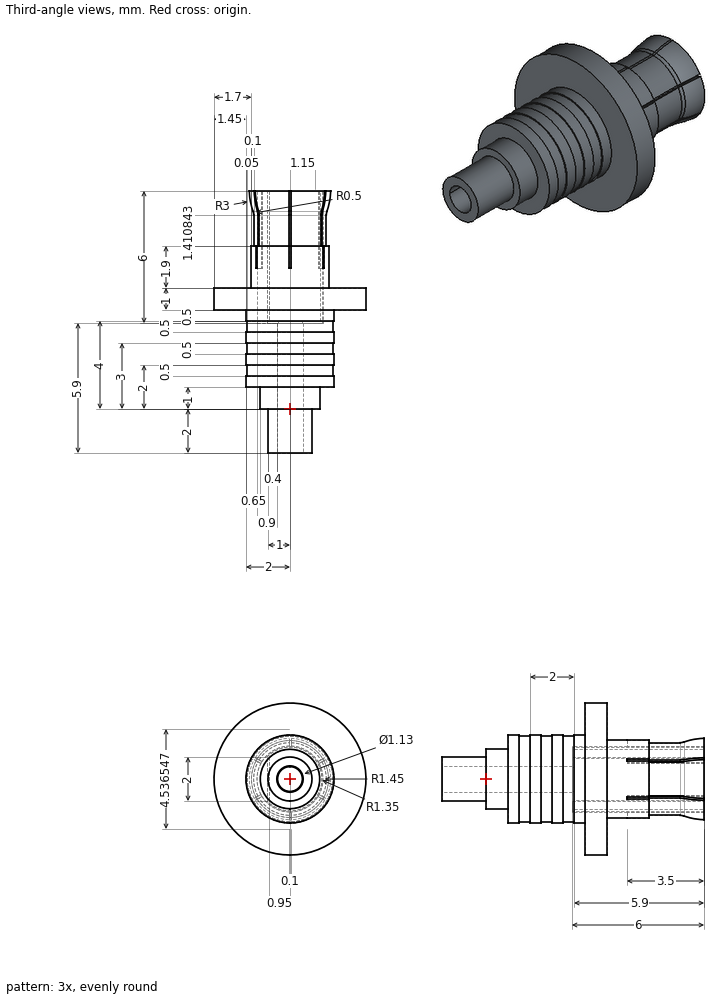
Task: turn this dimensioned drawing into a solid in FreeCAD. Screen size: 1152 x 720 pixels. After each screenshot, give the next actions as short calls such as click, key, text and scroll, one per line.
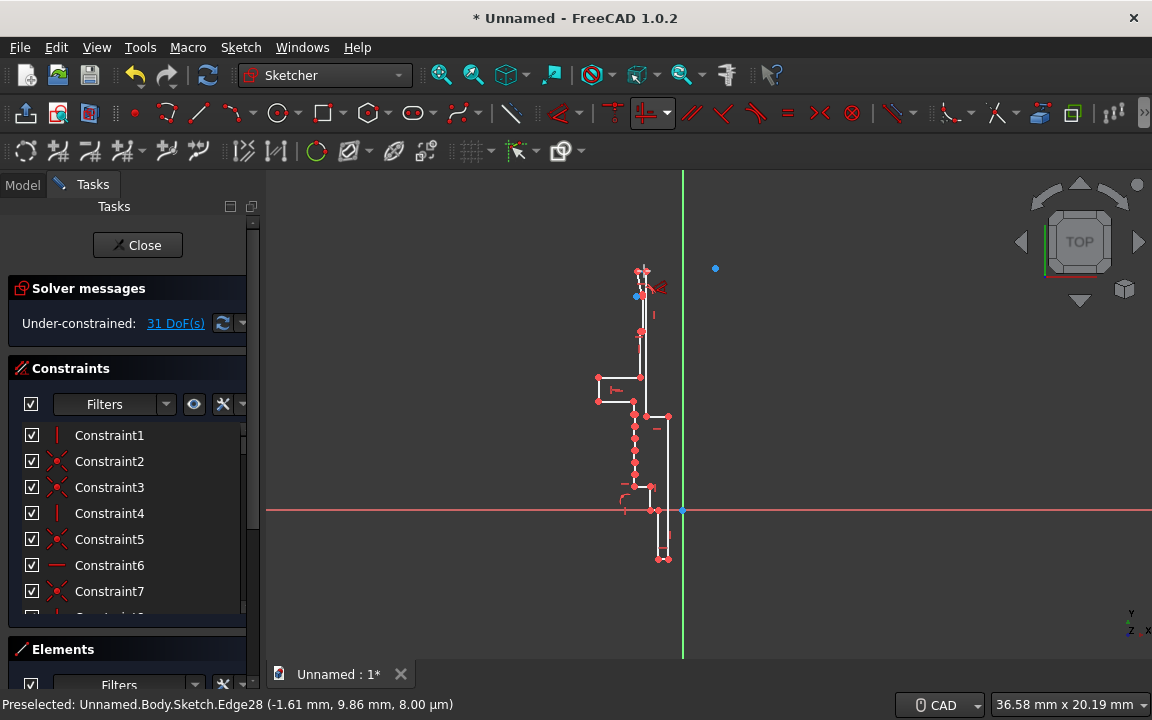
scroll(638, 279, up, 4)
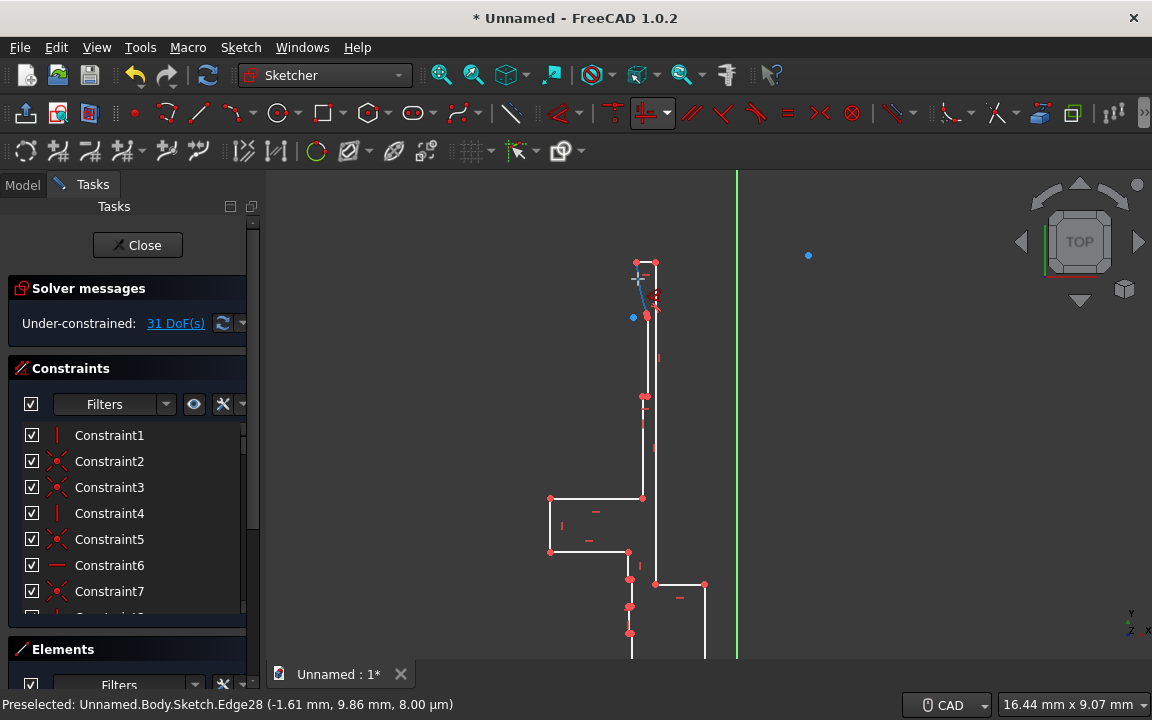
click(638, 278)
click(606, 282)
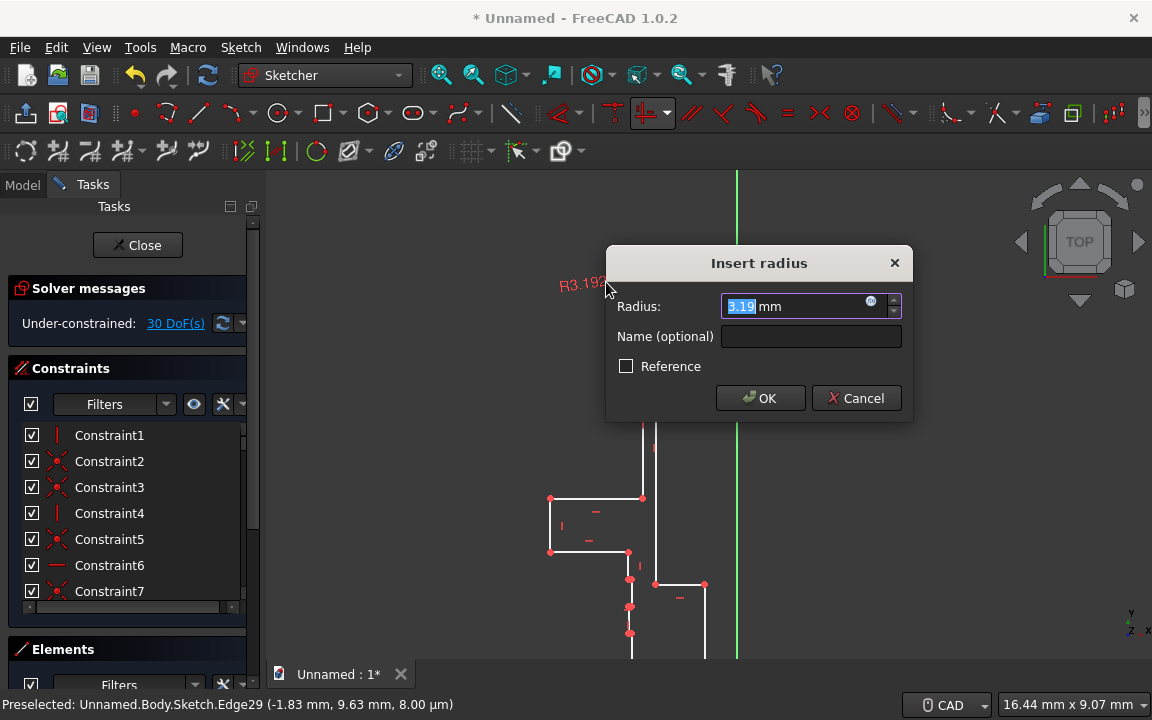
text(3)
key(Return)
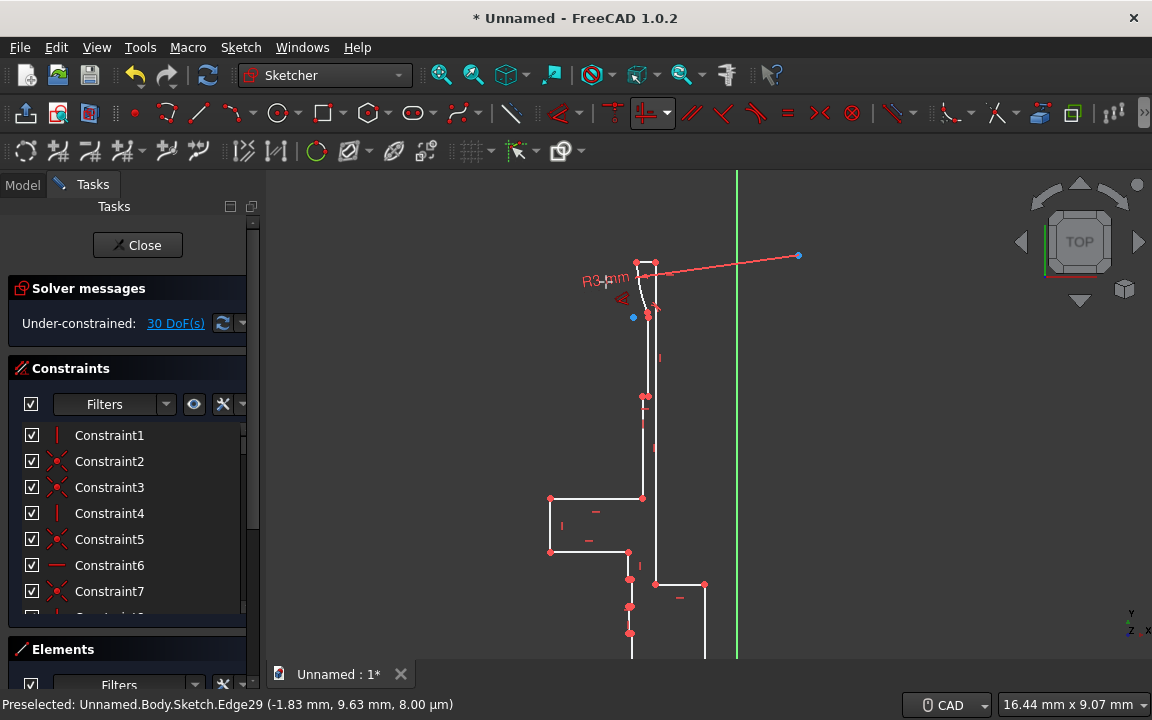
scroll(648, 315, up, 9)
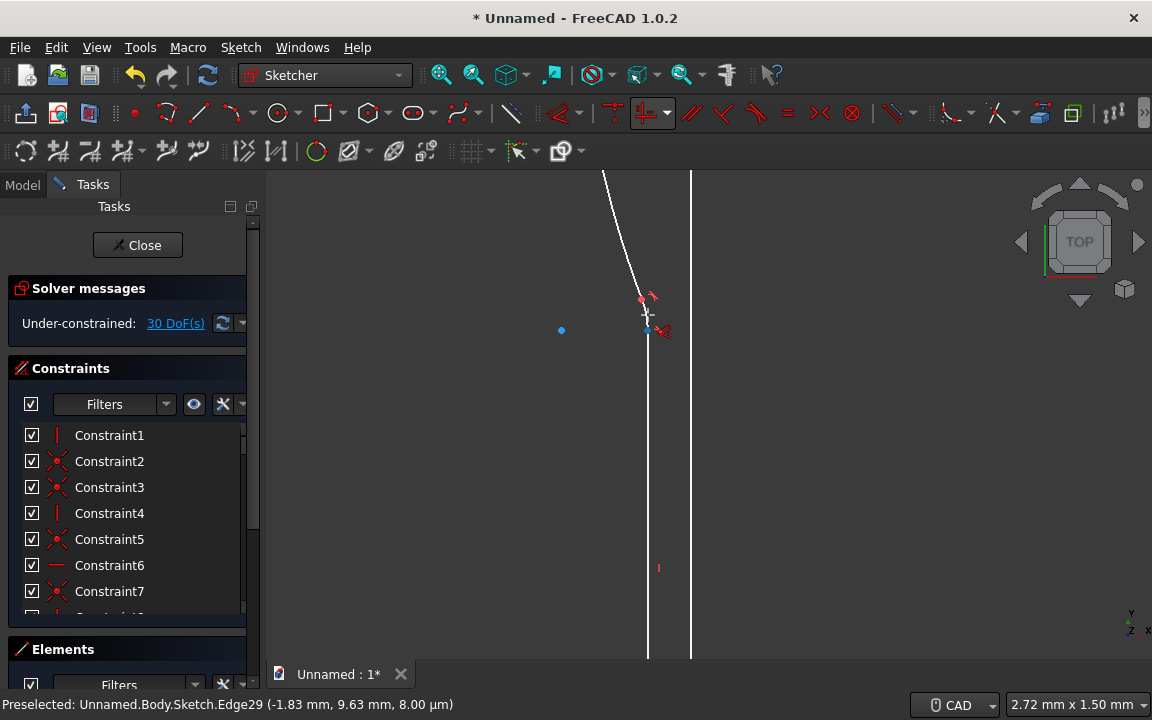
click(646, 314)
click(677, 308)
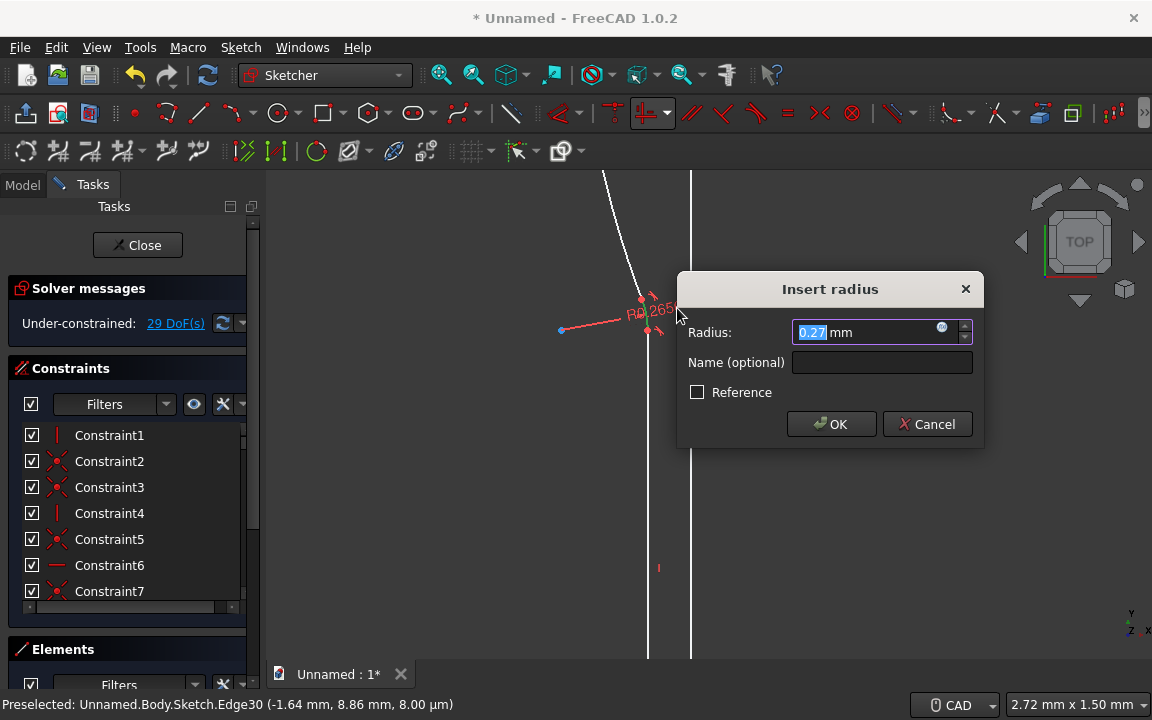
text(0.5)
key(Return)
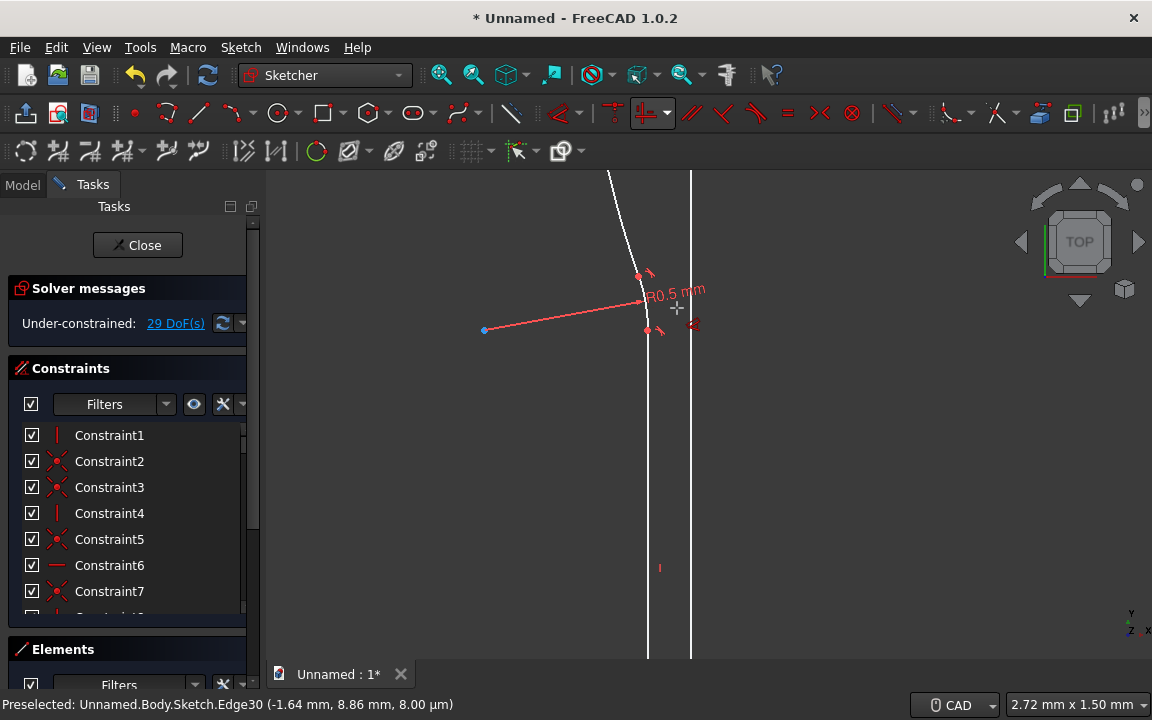
scroll(642, 294, down, 13)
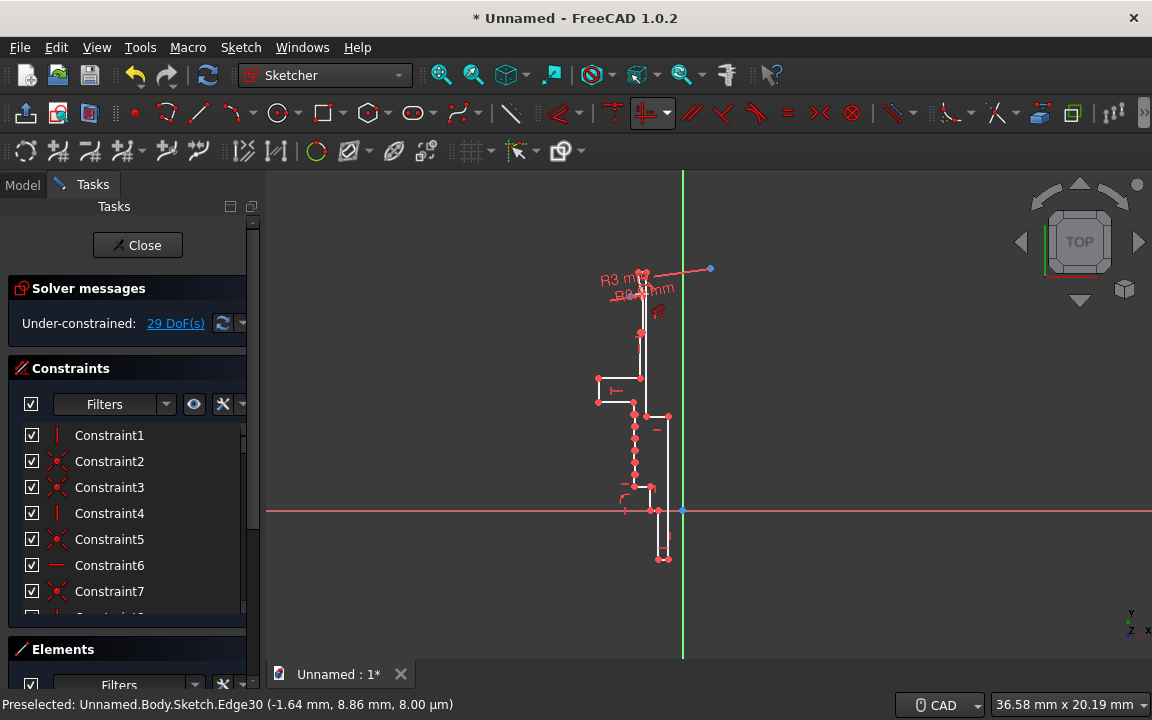
scroll(599, 386, up, 4)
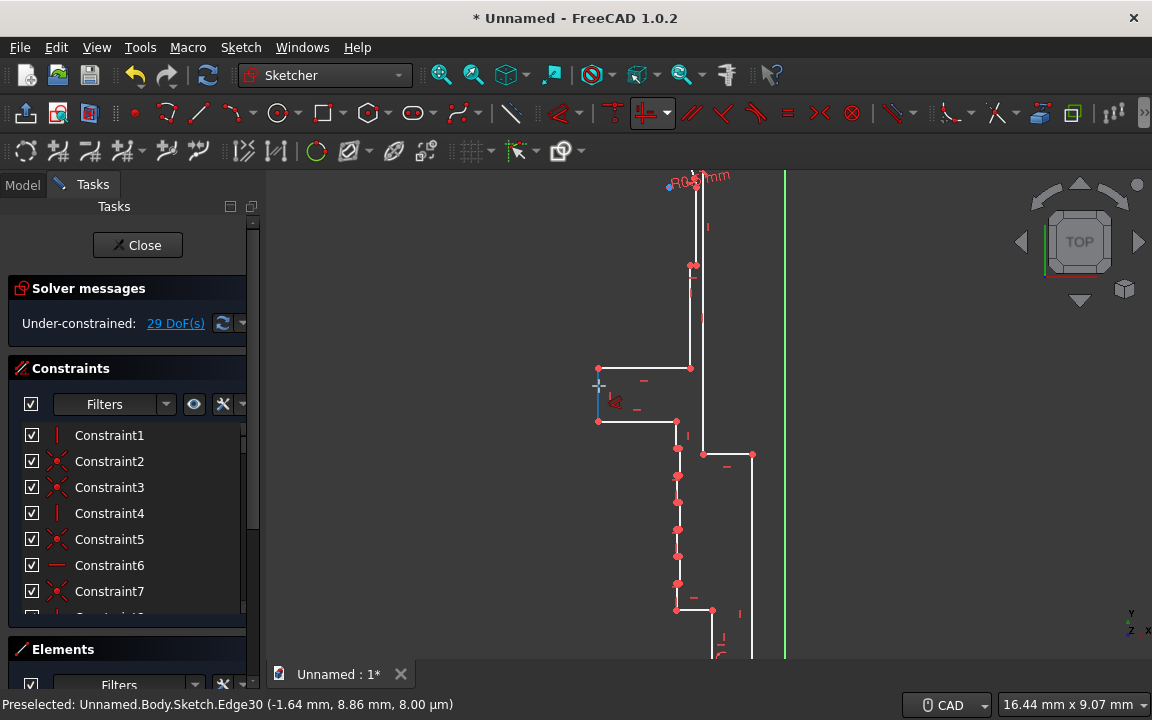
click(598, 384)
click(564, 395)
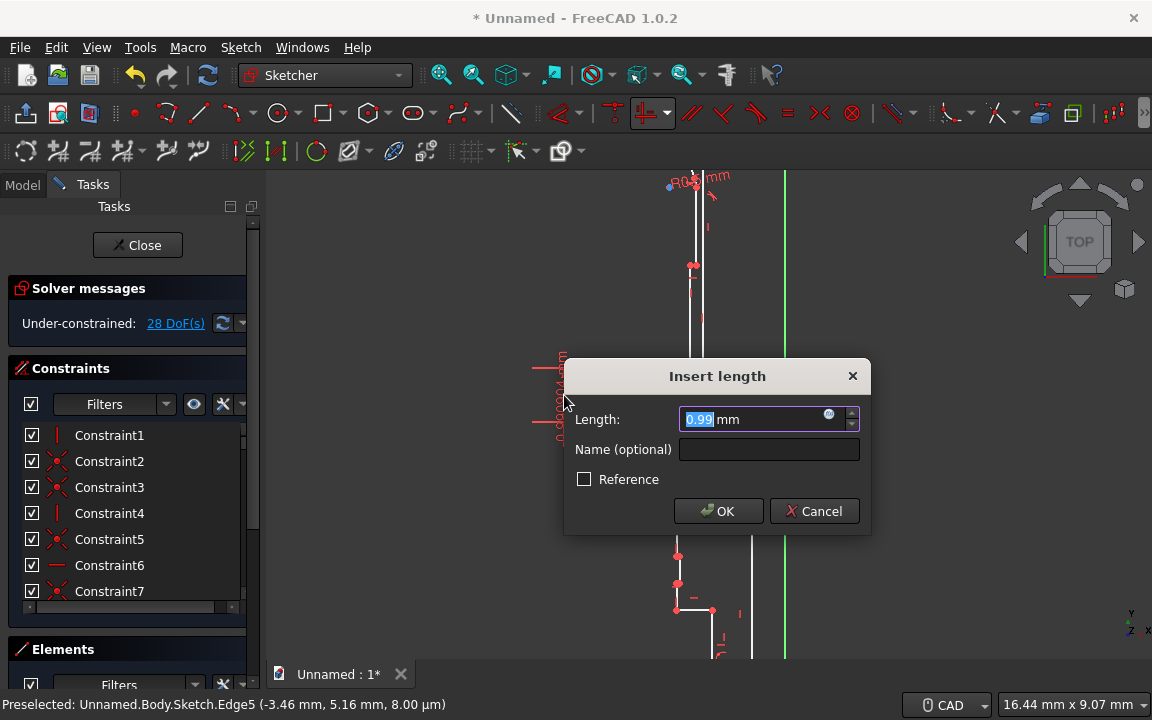
text(1)
key(Return)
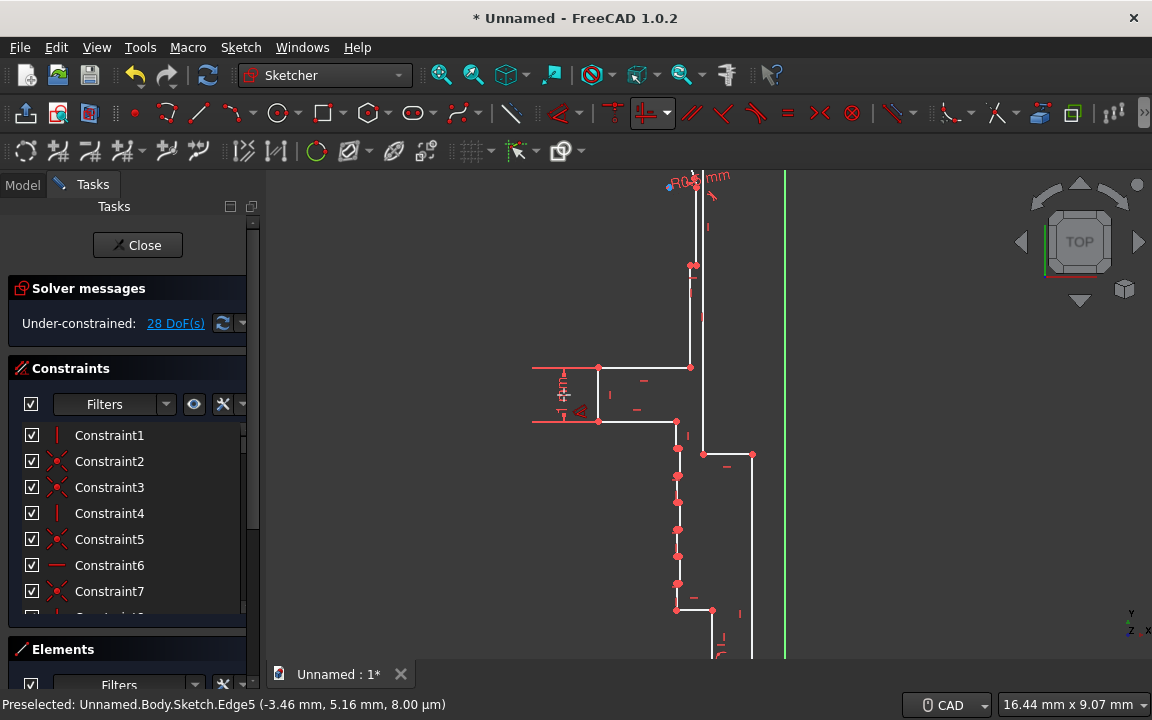
click(712, 626)
click(678, 625)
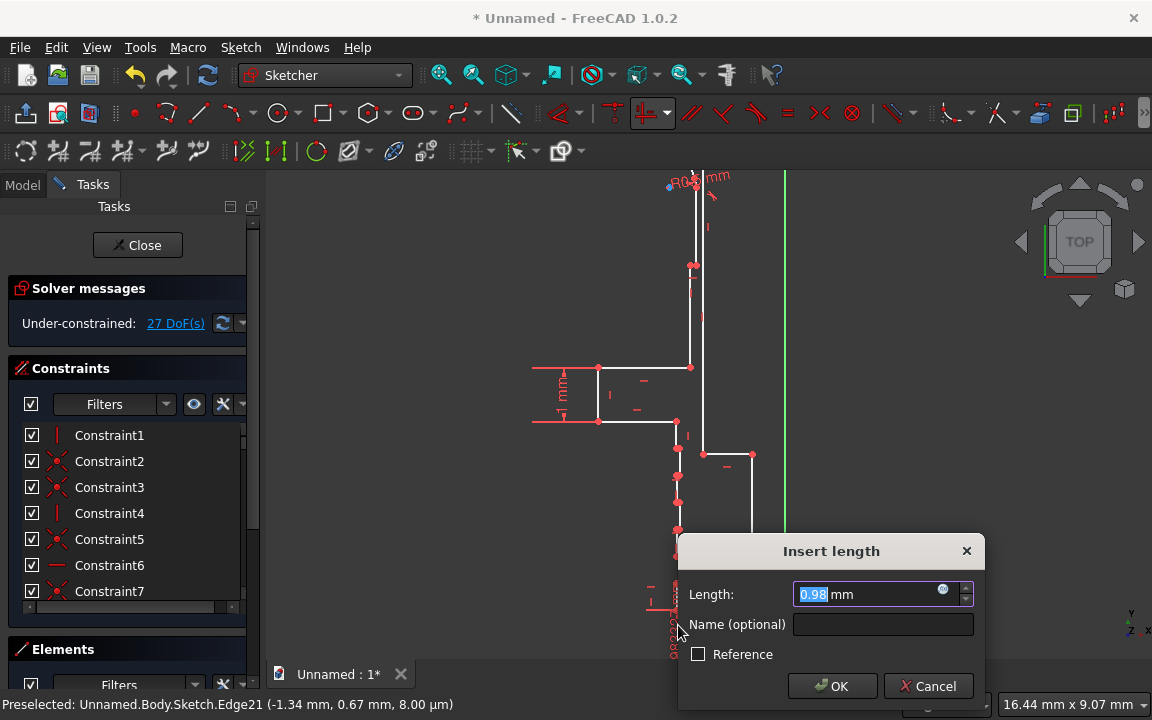
text(1)
key(Return)